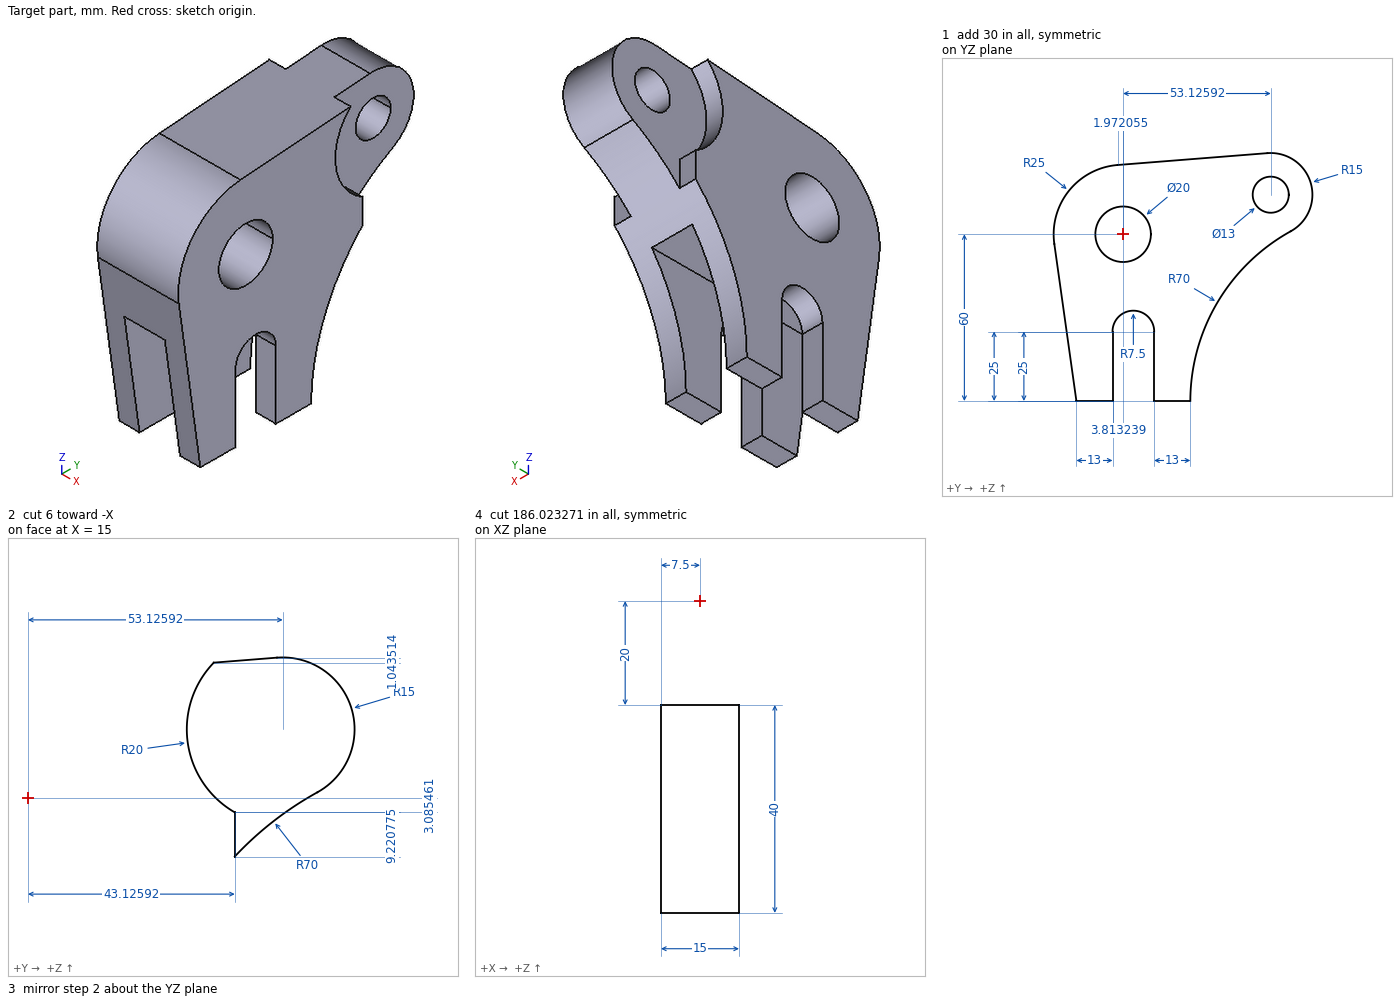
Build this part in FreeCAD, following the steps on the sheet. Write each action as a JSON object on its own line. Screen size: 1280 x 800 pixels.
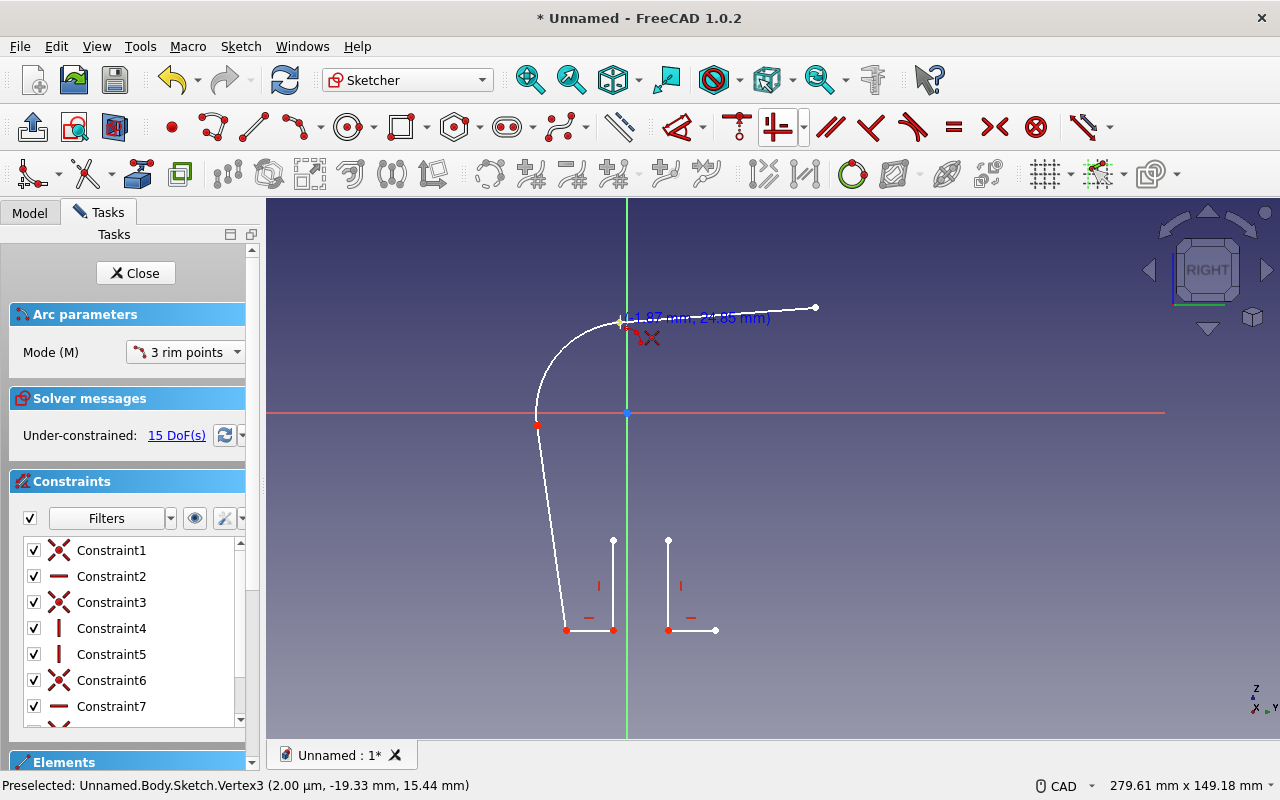
{"action": "left_click", "coordinate": [613, 541]}
{"action": "left_click", "coordinate": [668, 541]}
{"action": "left_click", "coordinate": [649, 514]}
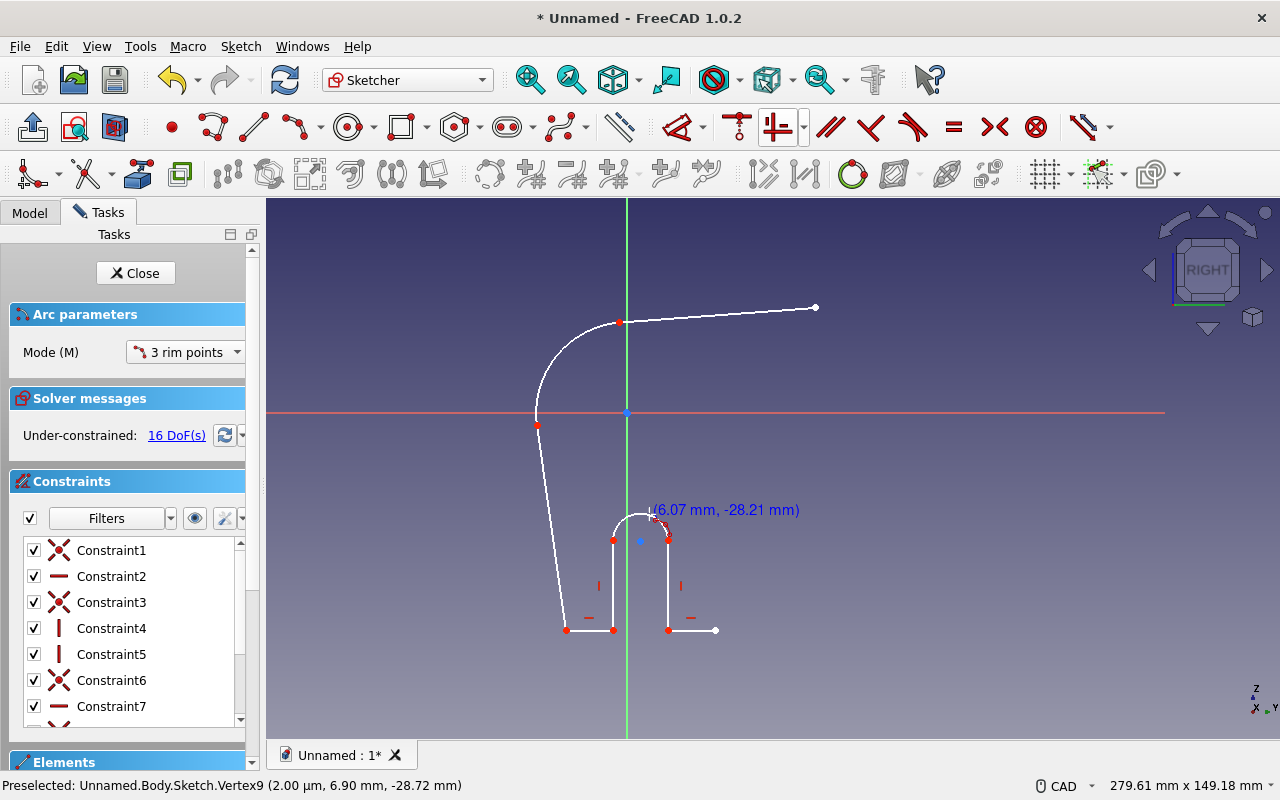
{"action": "left_click", "coordinate": [715, 631]}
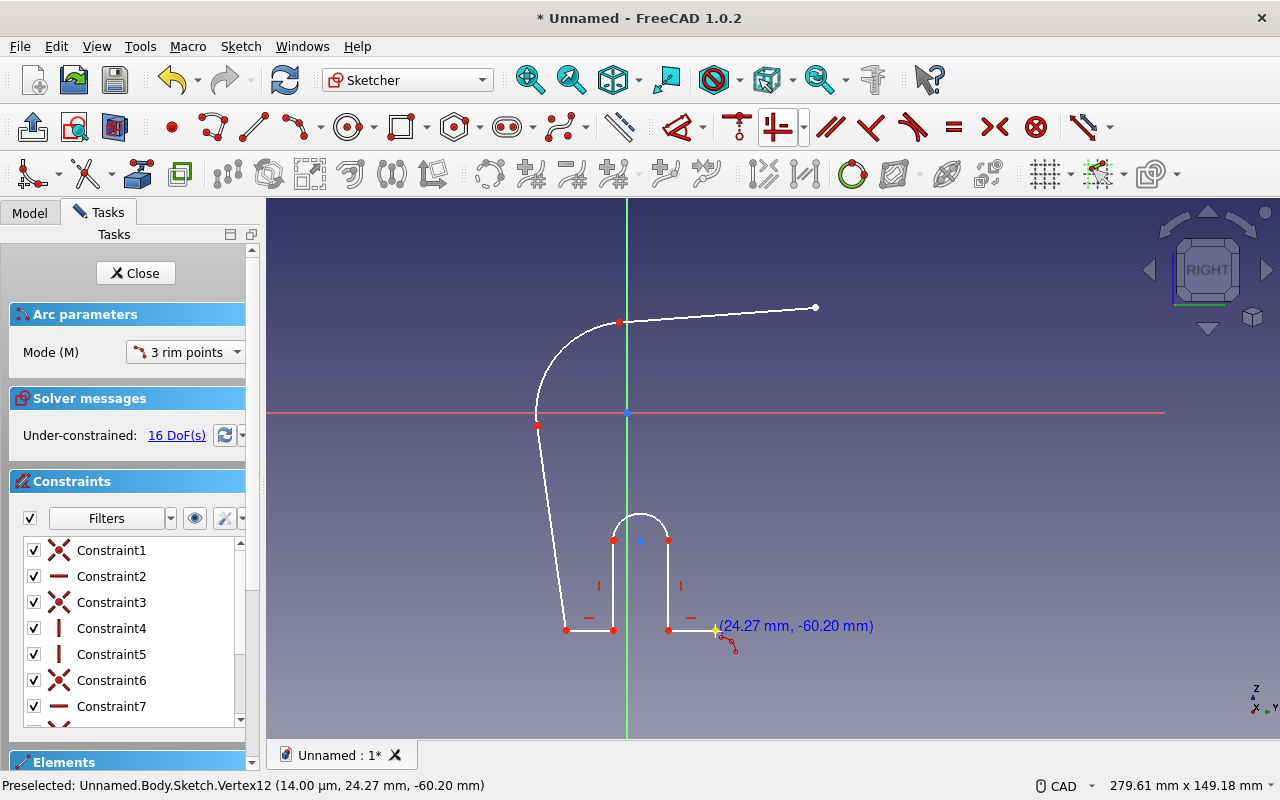
{"action": "scroll", "coordinate": [846, 409], "scroll_direction": "up", "scroll_amount": 7}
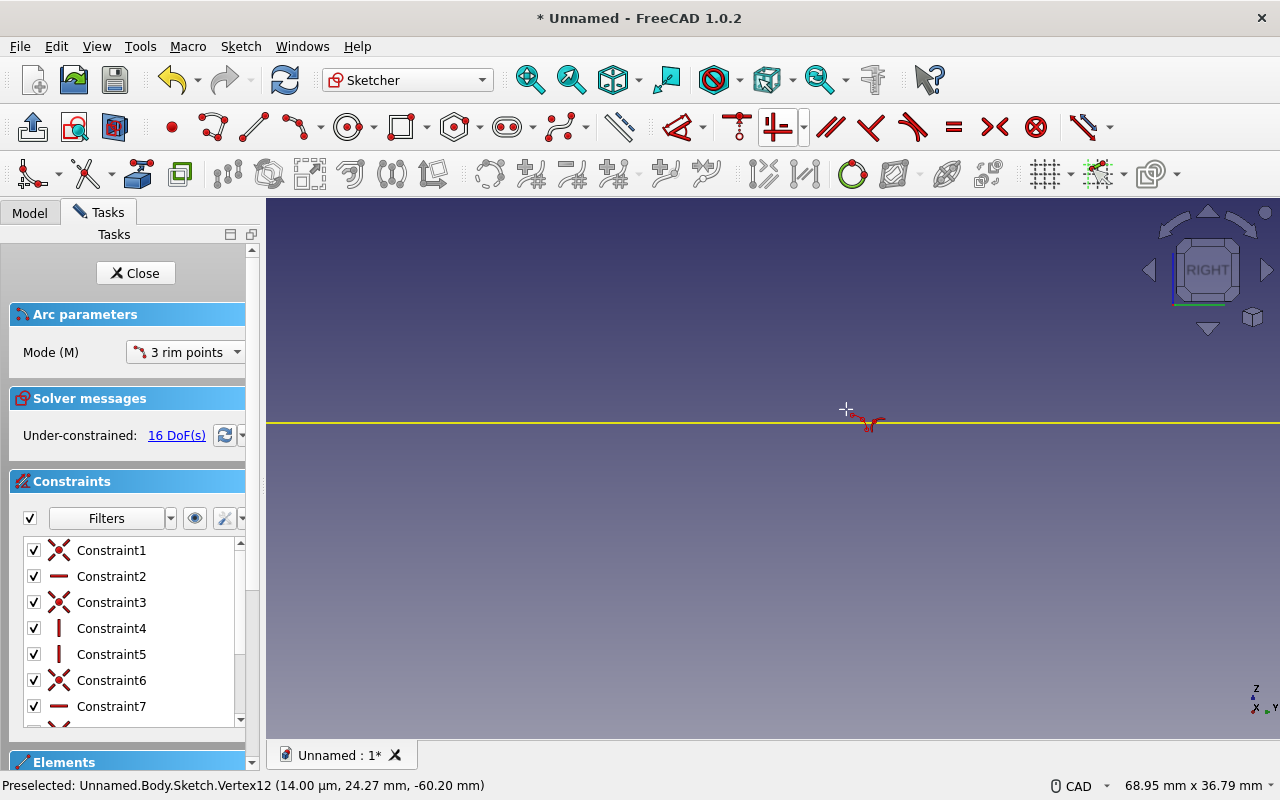
{"action": "left_click", "coordinate": [844, 407]}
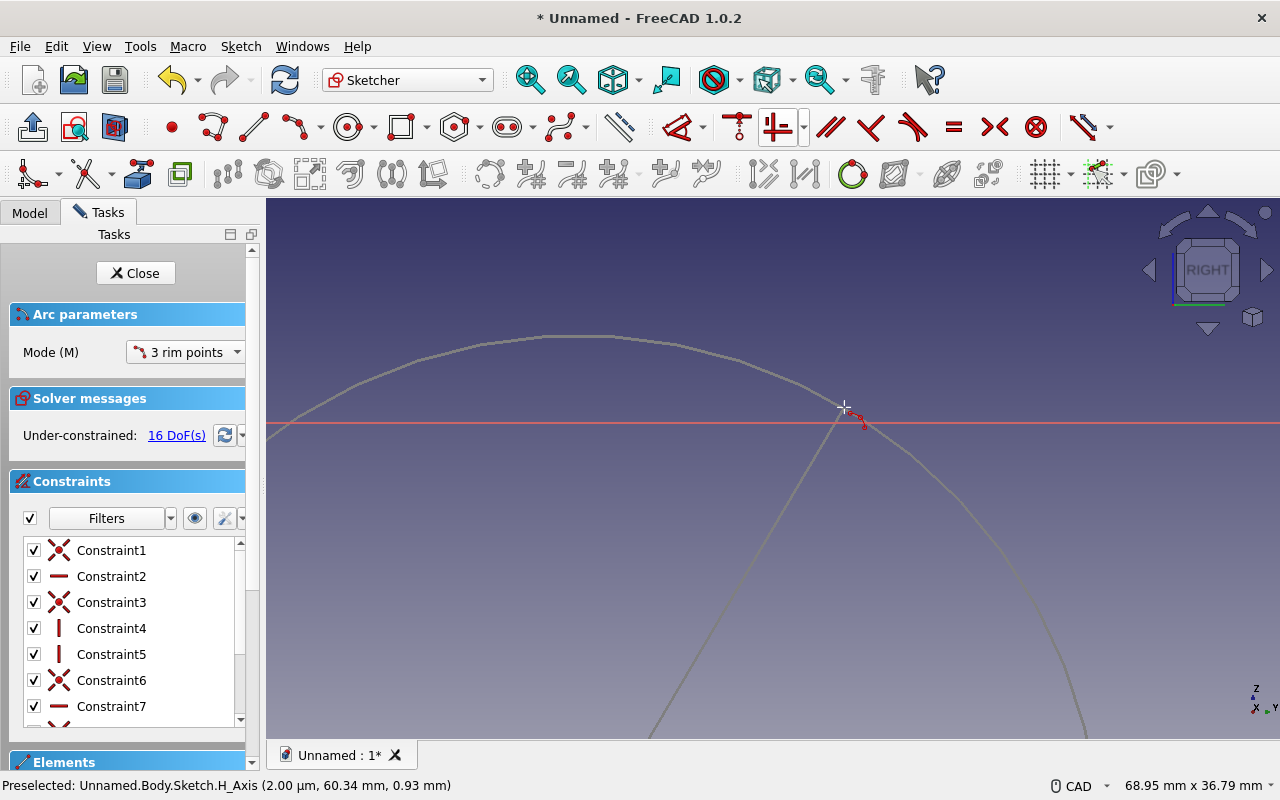
{"action": "scroll", "coordinate": [847, 409], "scroll_direction": "down", "scroll_amount": 7}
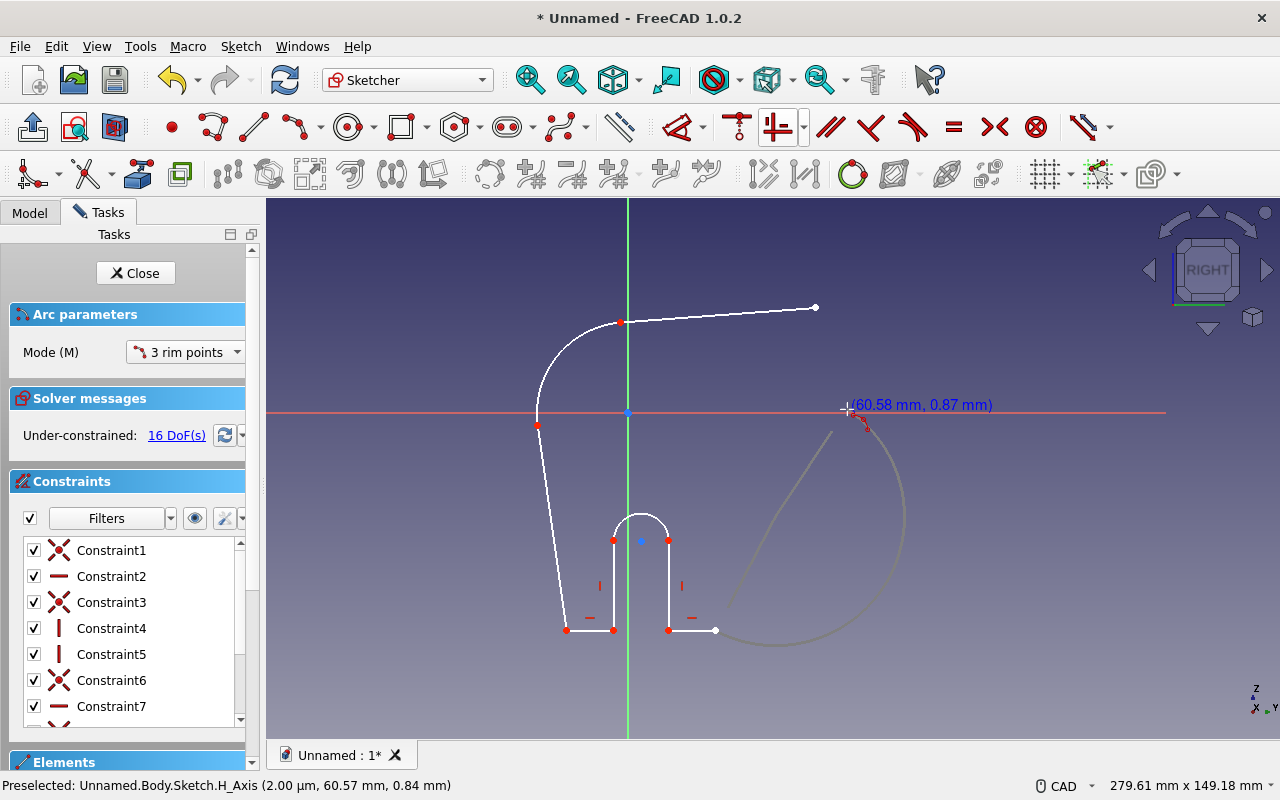
{"action": "left_click", "coordinate": [751, 502]}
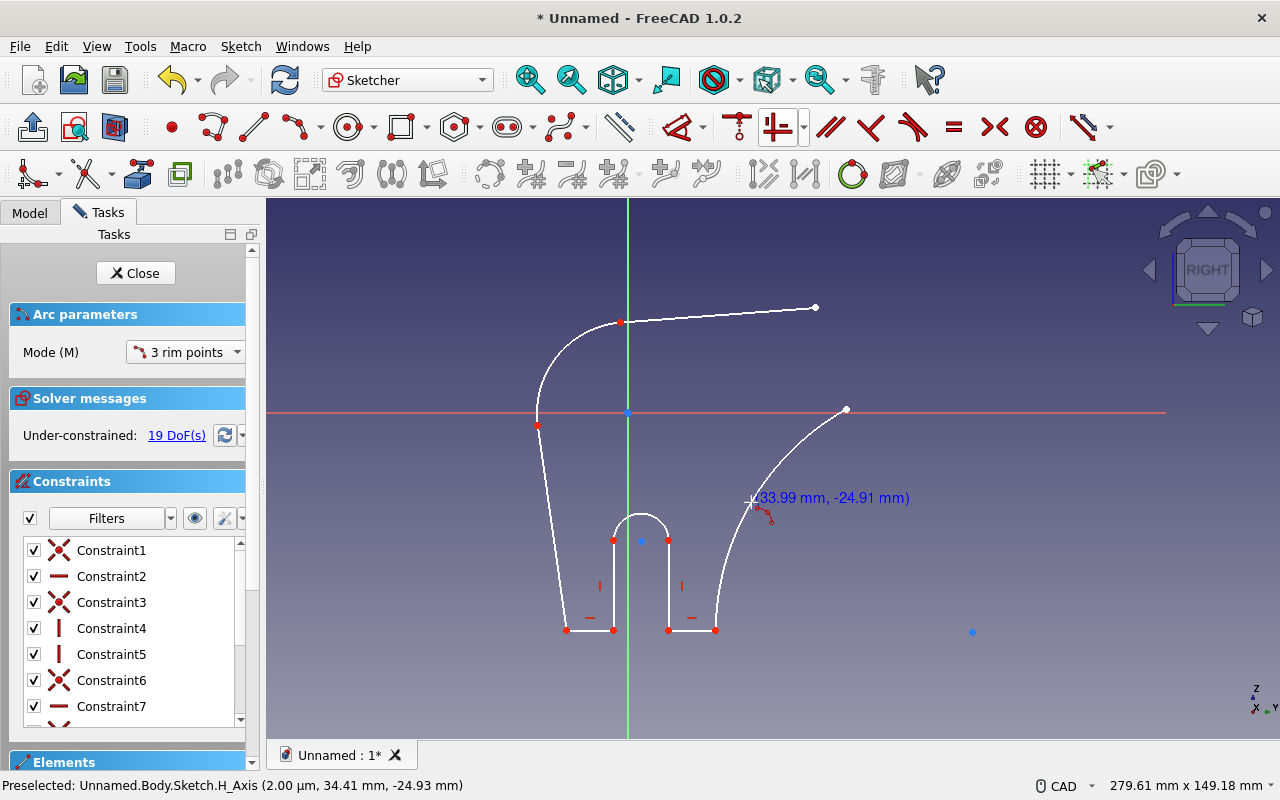
{"action": "scroll", "coordinate": [847, 409], "scroll_direction": "up", "scroll_amount": 7}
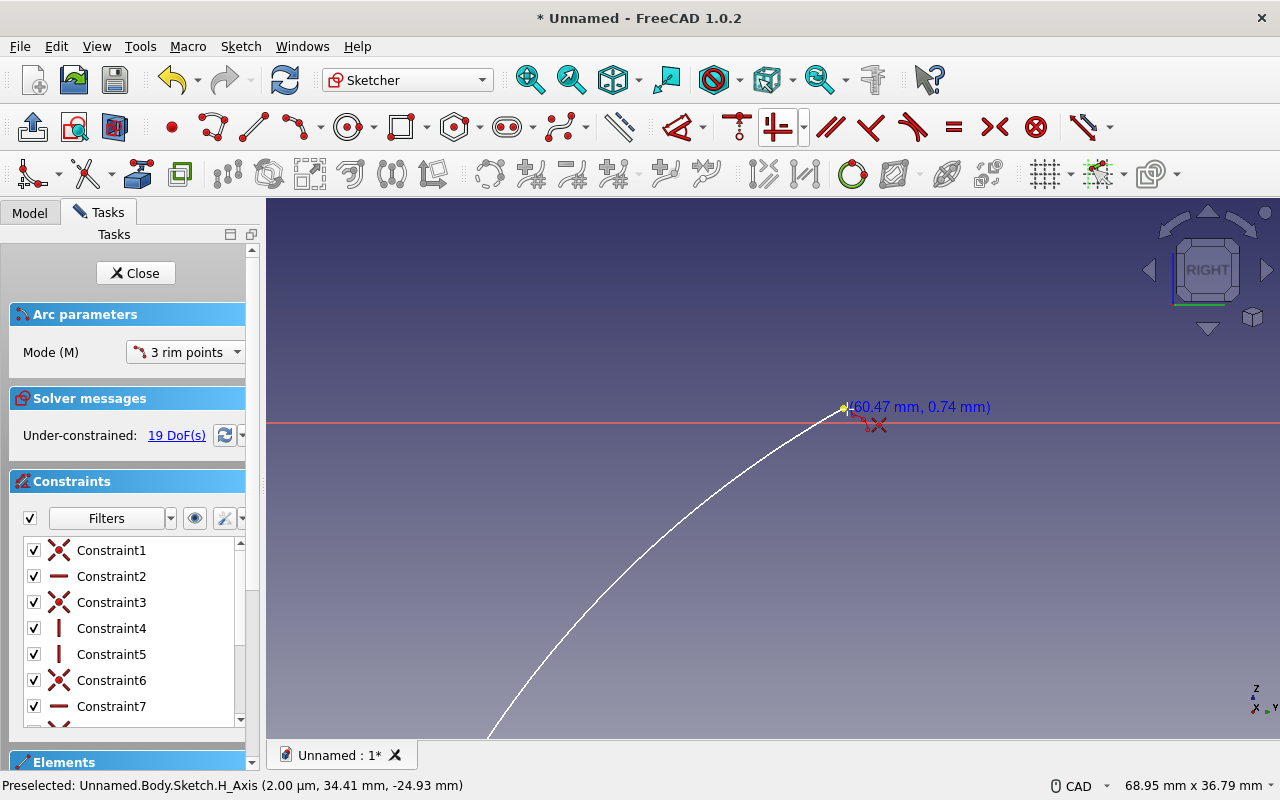
{"action": "left_click", "coordinate": [844, 408]}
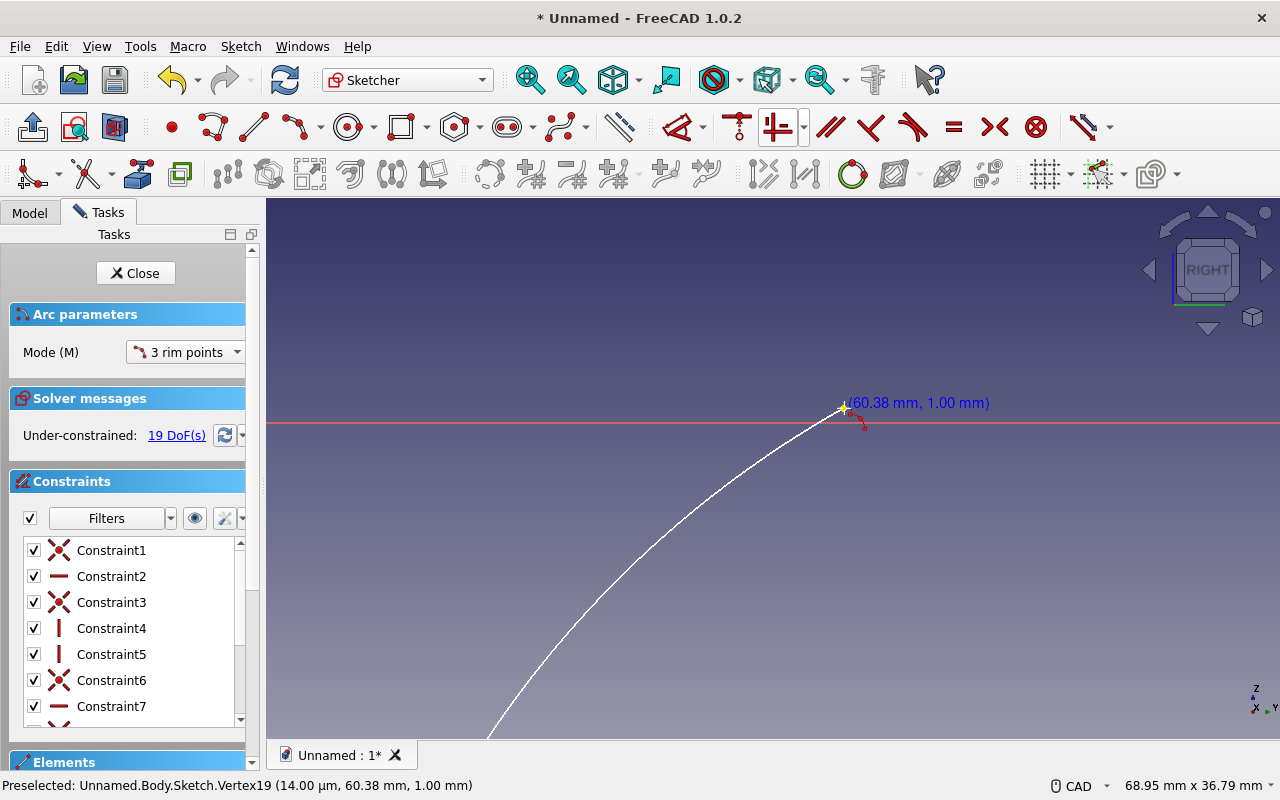
{"action": "scroll", "coordinate": [847, 409], "scroll_direction": "down", "scroll_amount": 7}